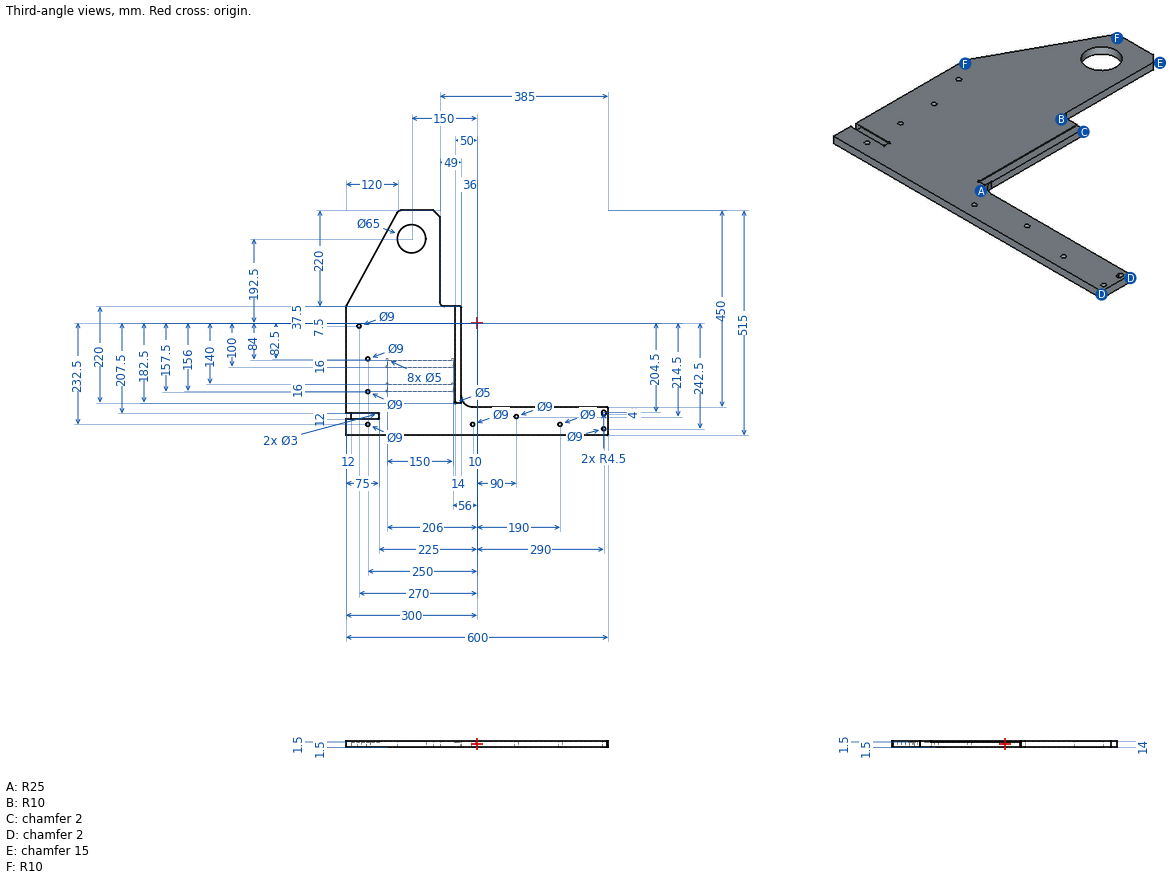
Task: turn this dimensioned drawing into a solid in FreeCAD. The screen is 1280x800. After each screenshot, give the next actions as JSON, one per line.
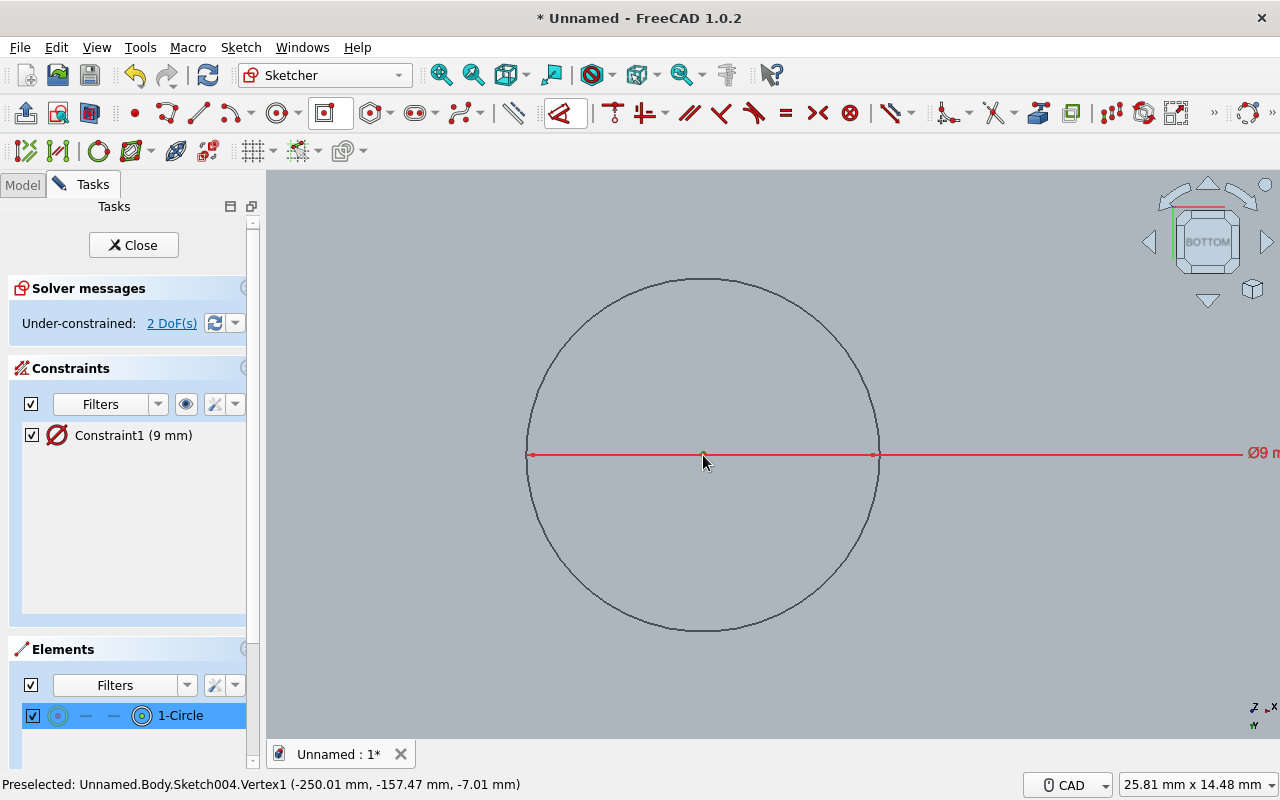
{"action": "left_click", "coordinate": [582, 114]}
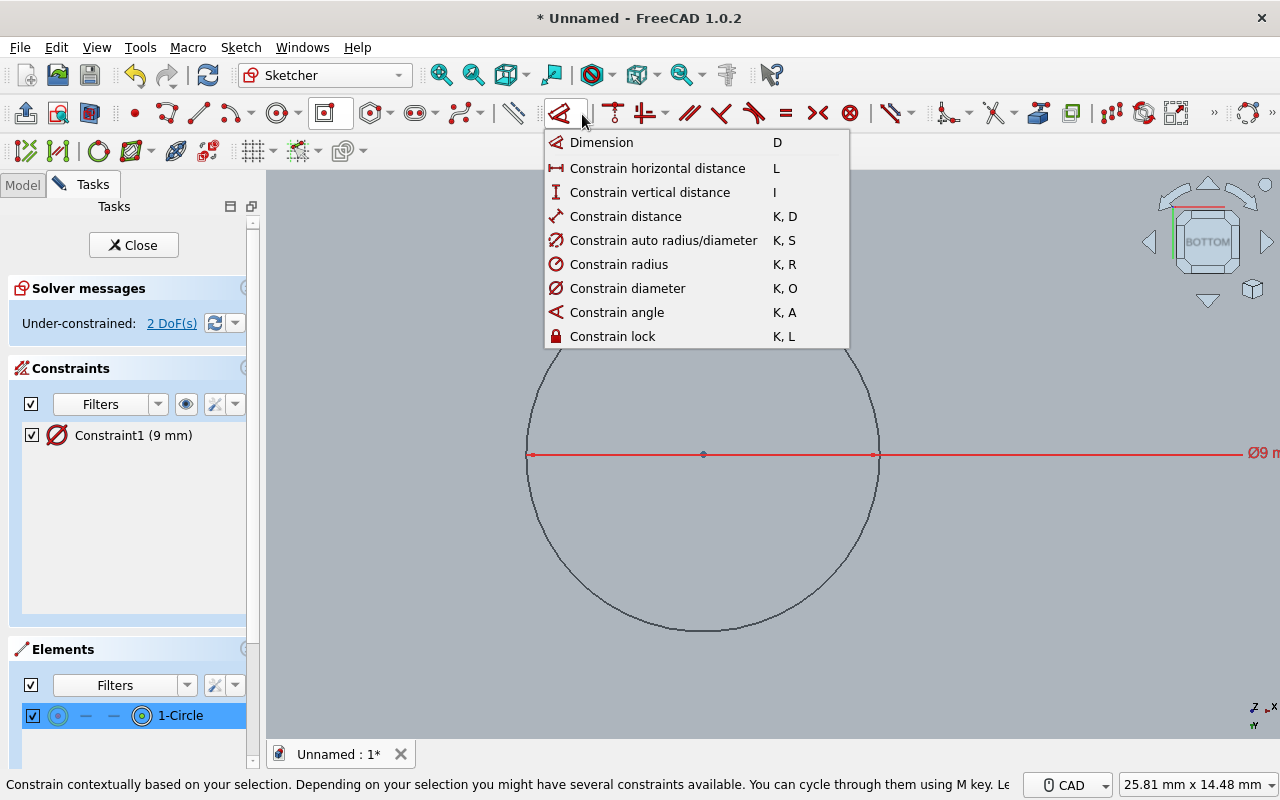
{"action": "left_click", "coordinate": [697, 168]}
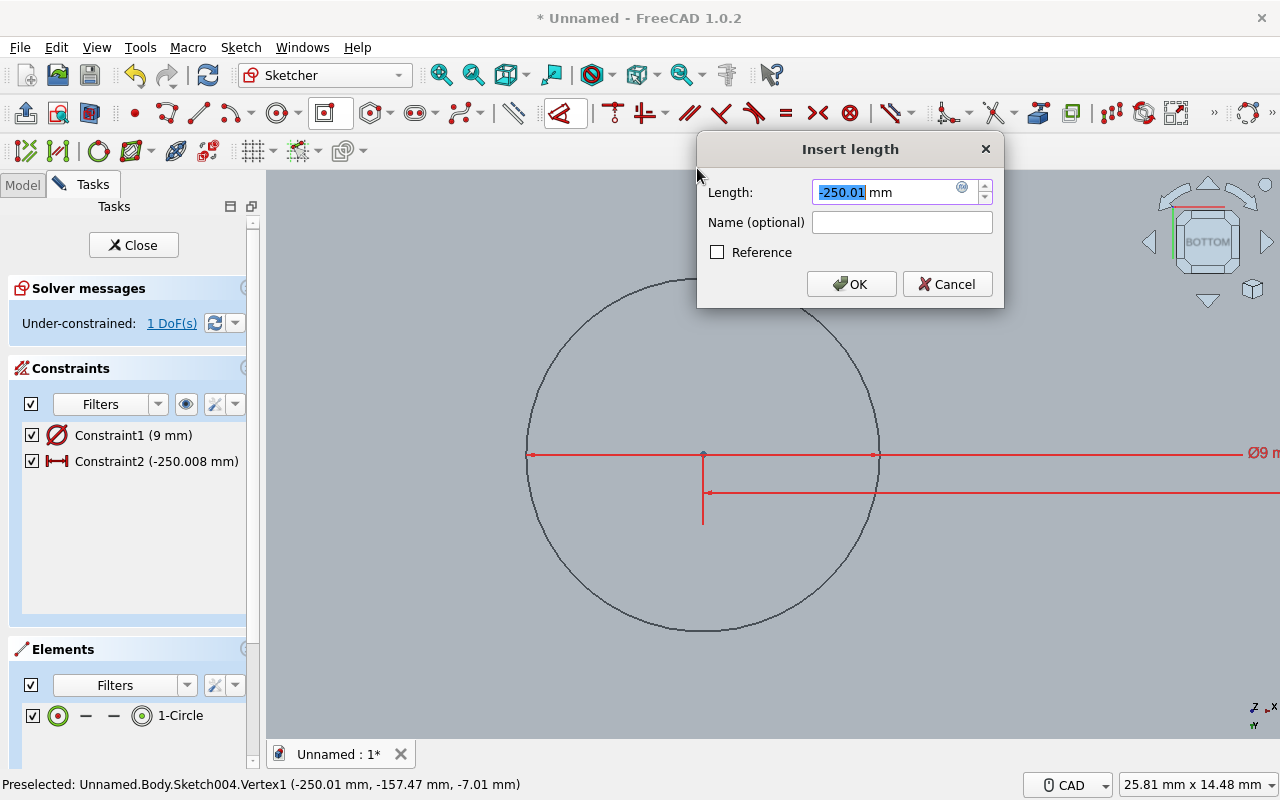
{"action": "type", "text": "-250"}
{"action": "key", "text": "Return"}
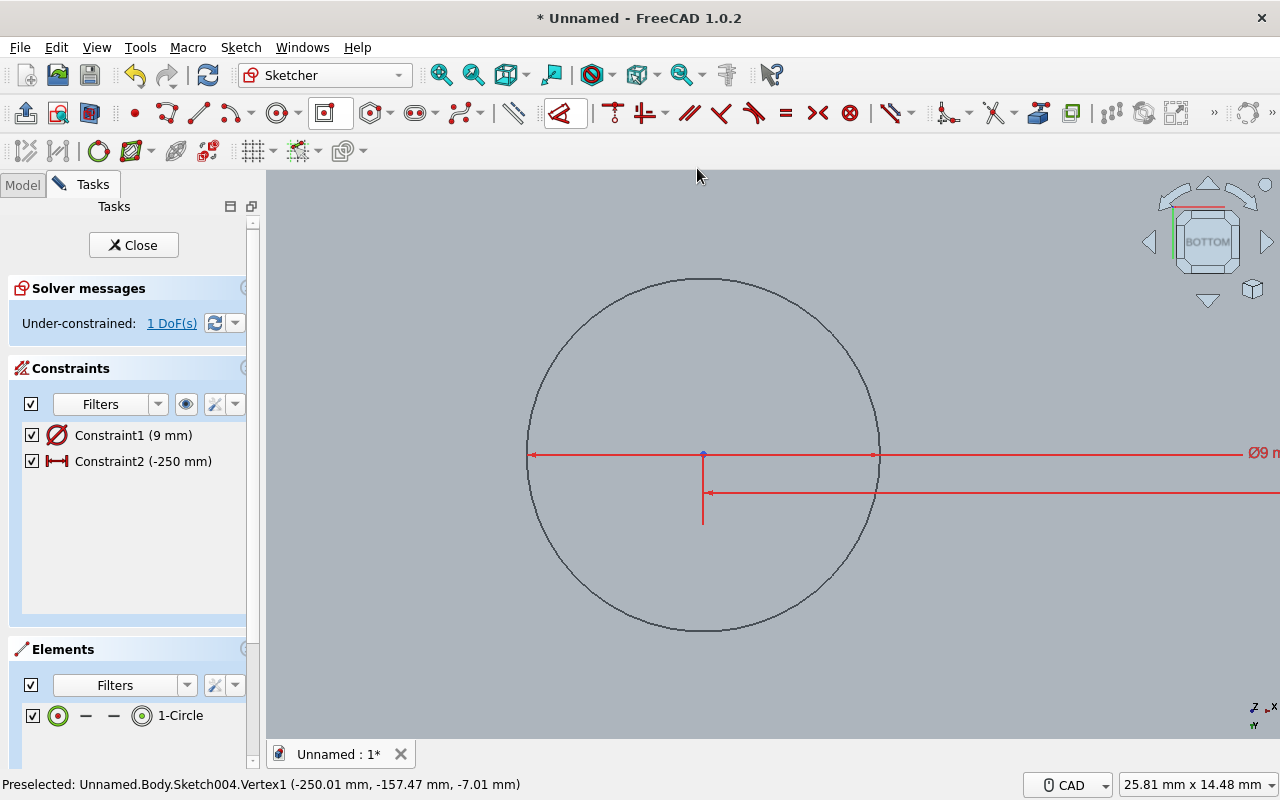
{"action": "left_click", "coordinate": [703, 455]}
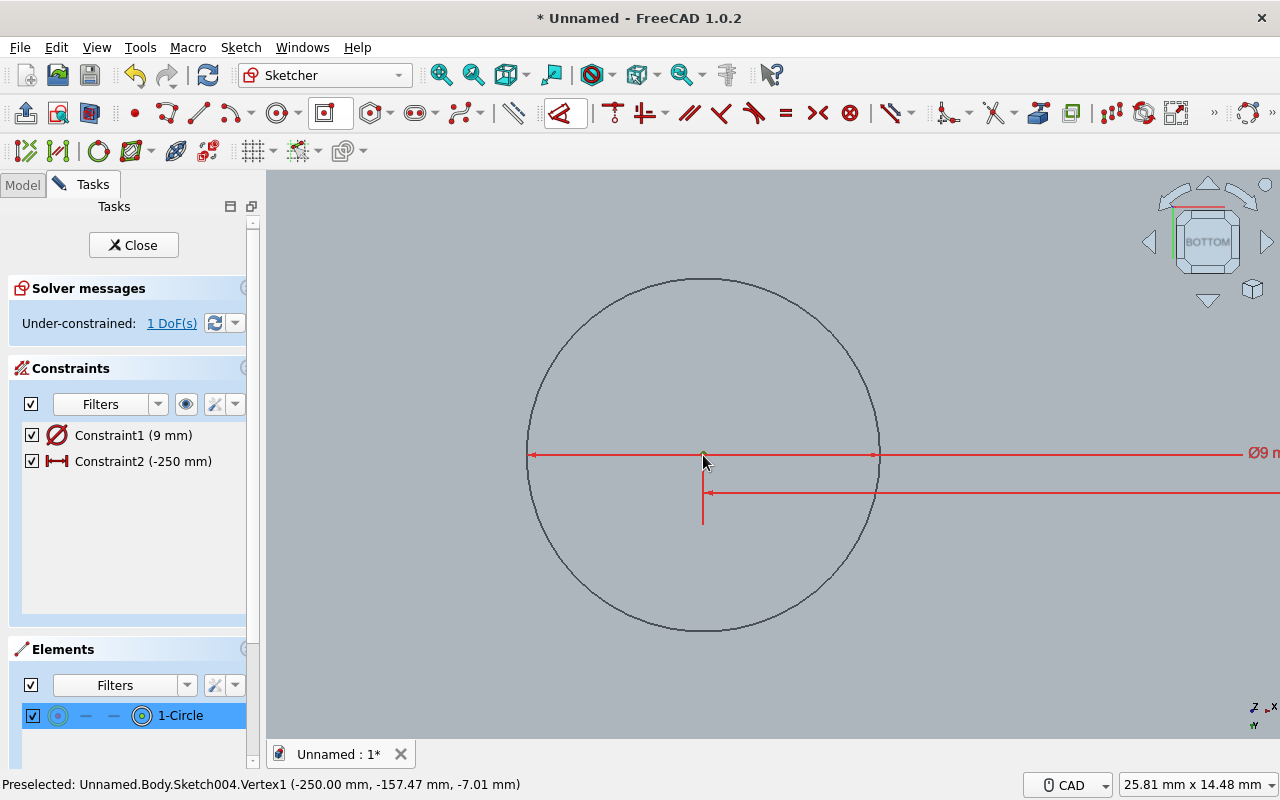
{"action": "left_click", "coordinate": [582, 114]}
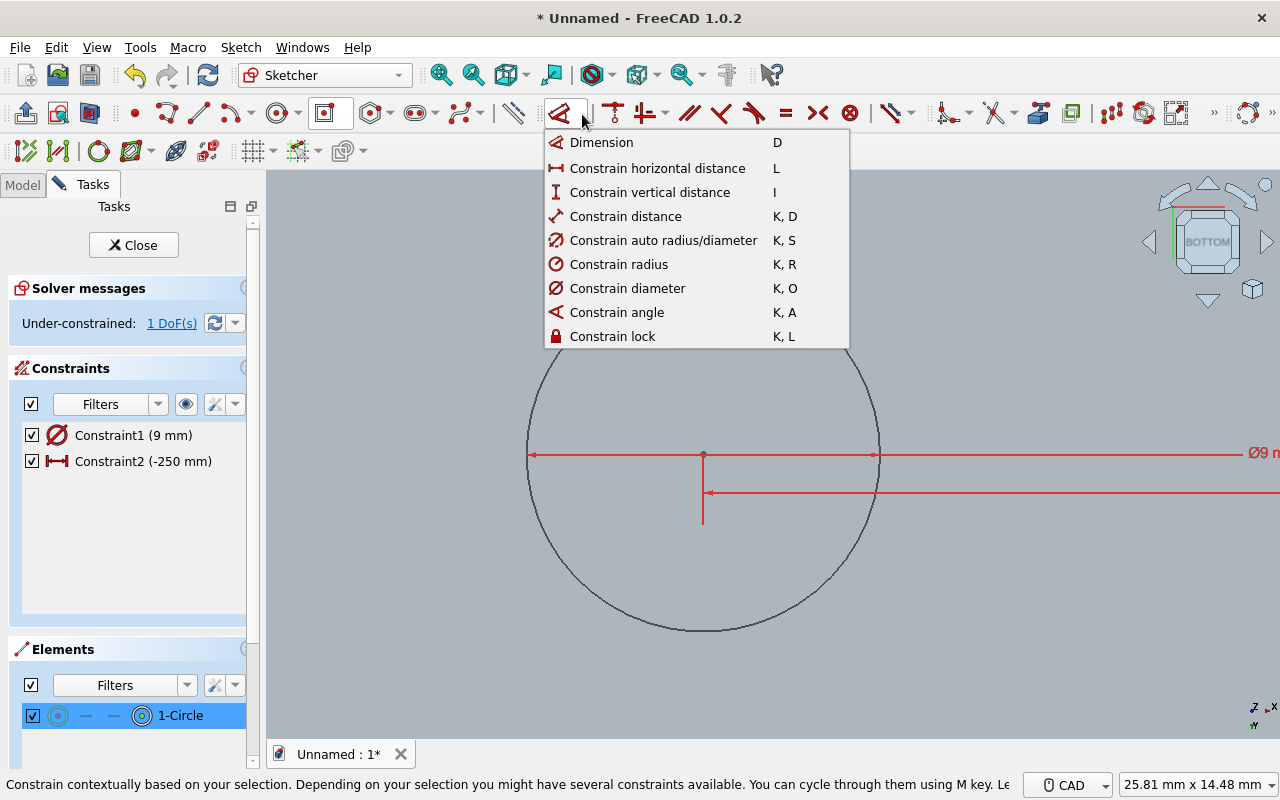
{"action": "left_click", "coordinate": [697, 192]}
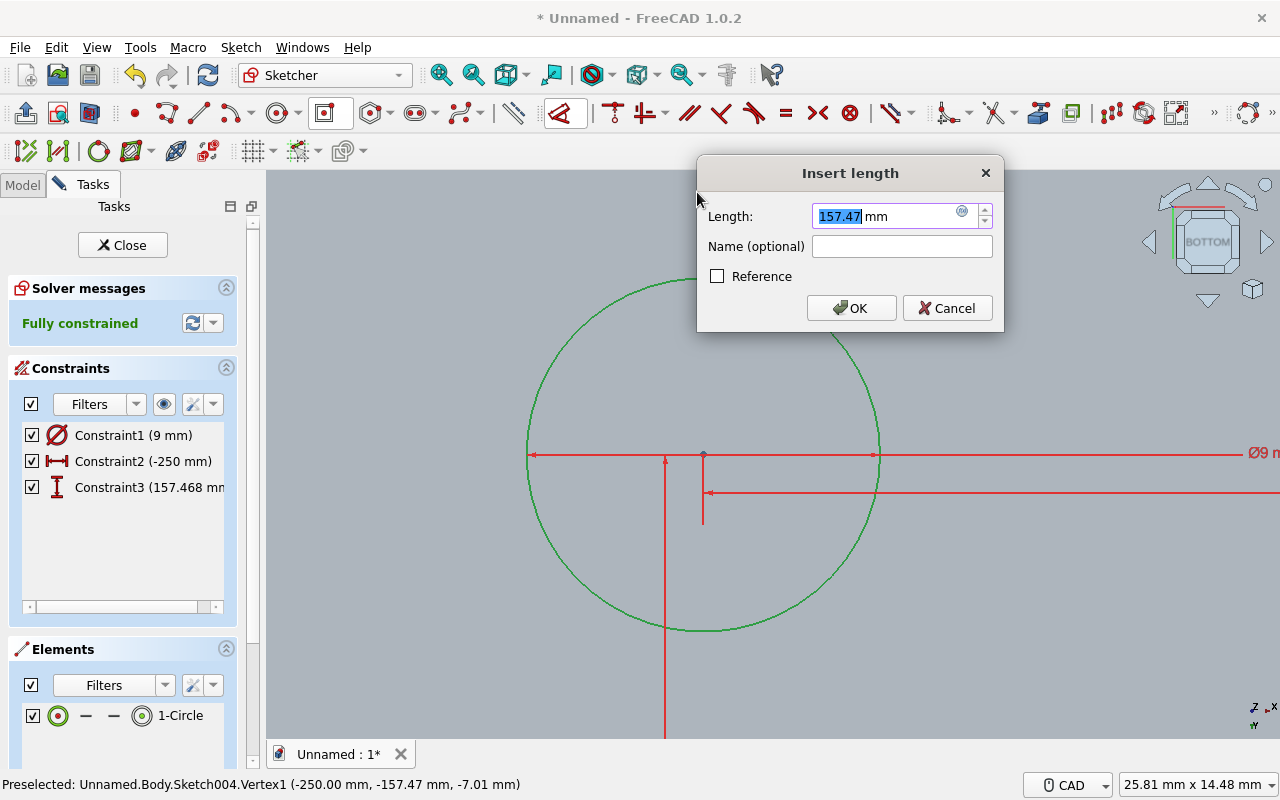
{"action": "type", "text": "157.5"}
{"action": "key", "text": "Return"}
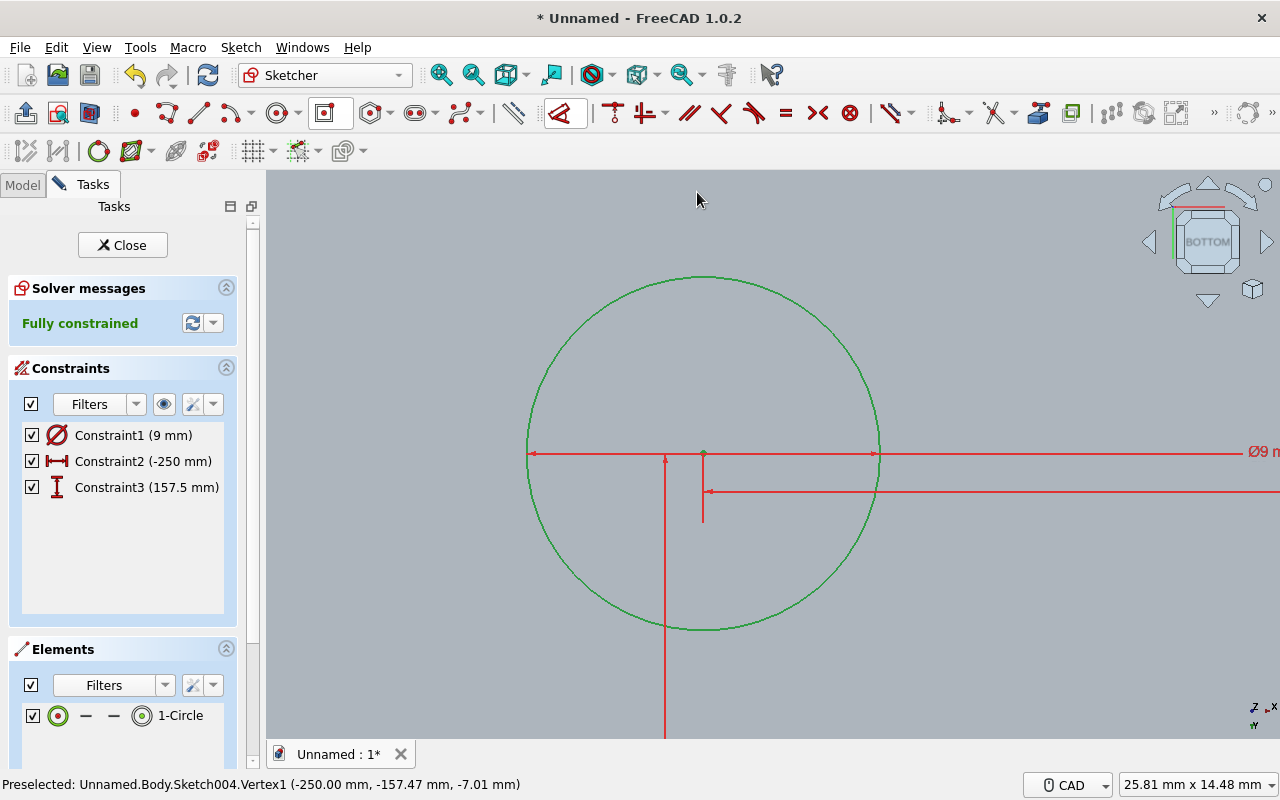
{"action": "left_click", "coordinate": [123, 245]}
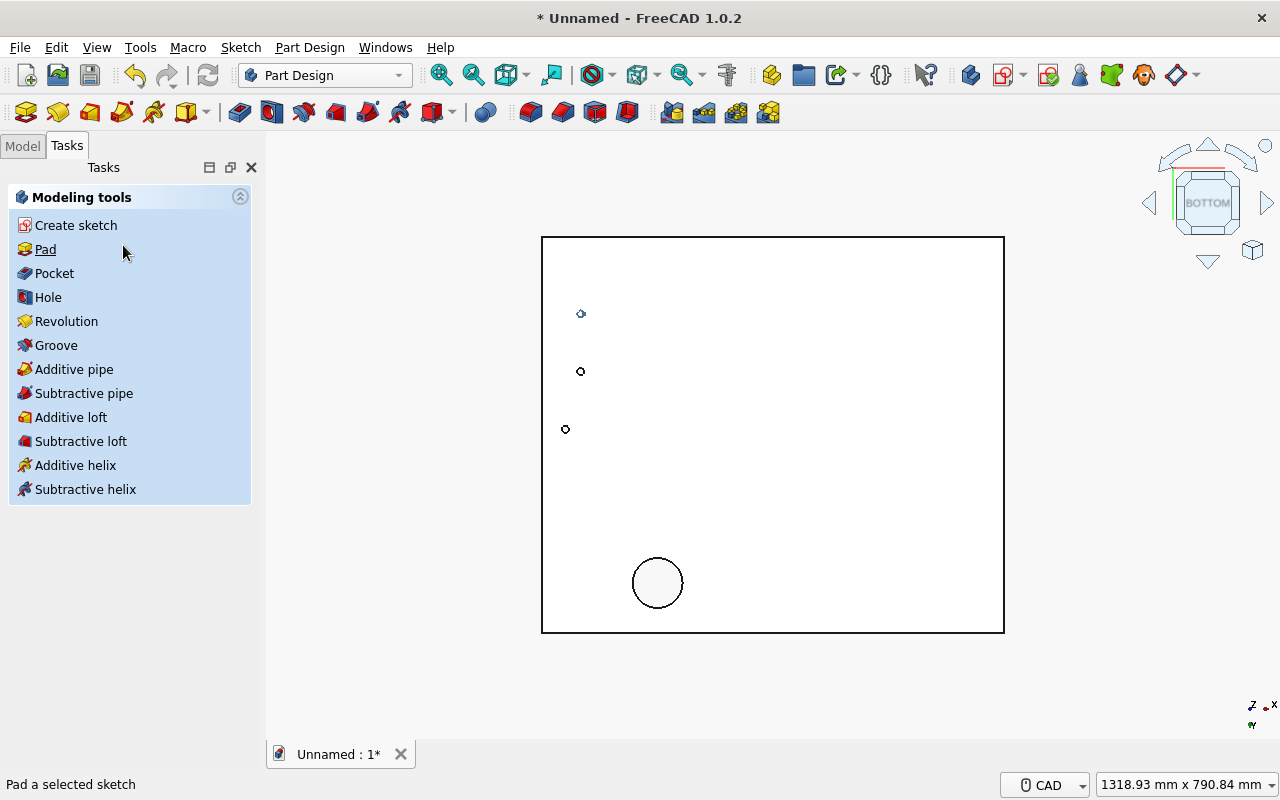
{"action": "left_click", "coordinate": [240, 112]}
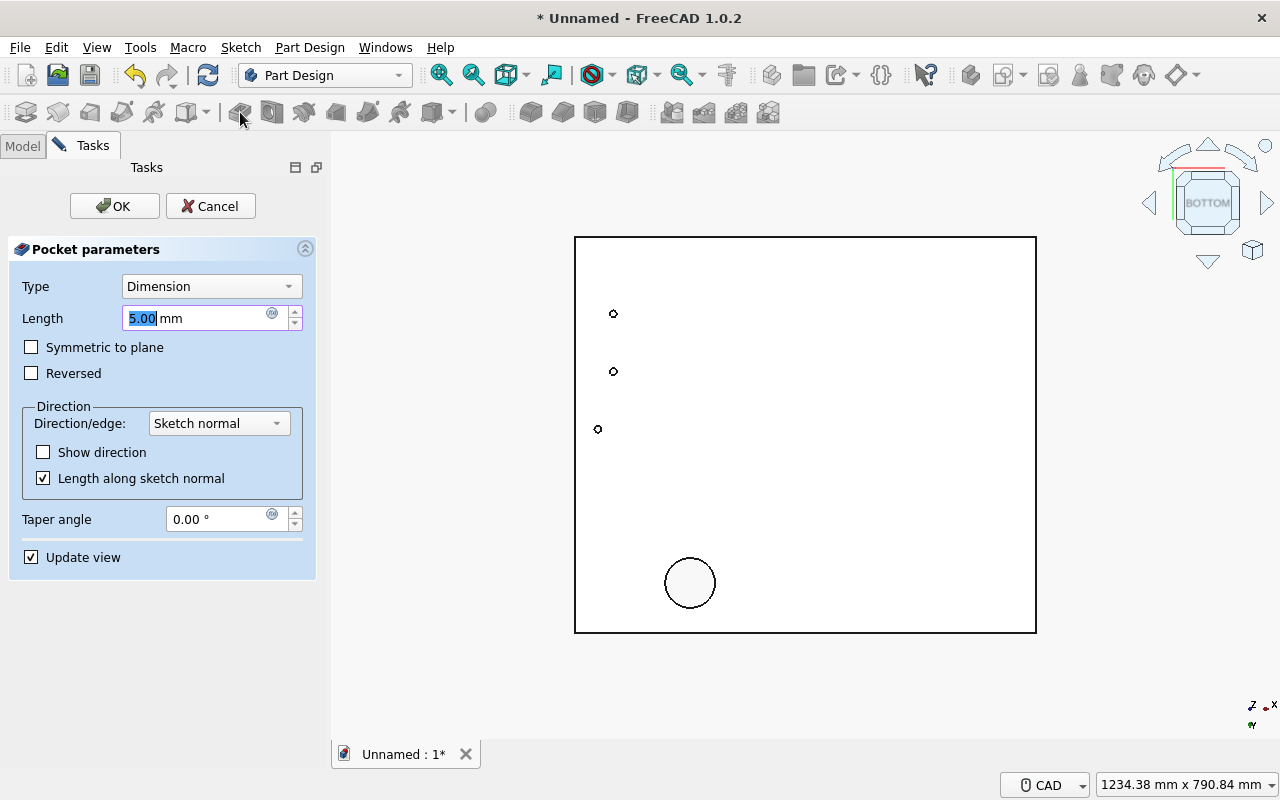
{"action": "left_click", "coordinate": [212, 286]}